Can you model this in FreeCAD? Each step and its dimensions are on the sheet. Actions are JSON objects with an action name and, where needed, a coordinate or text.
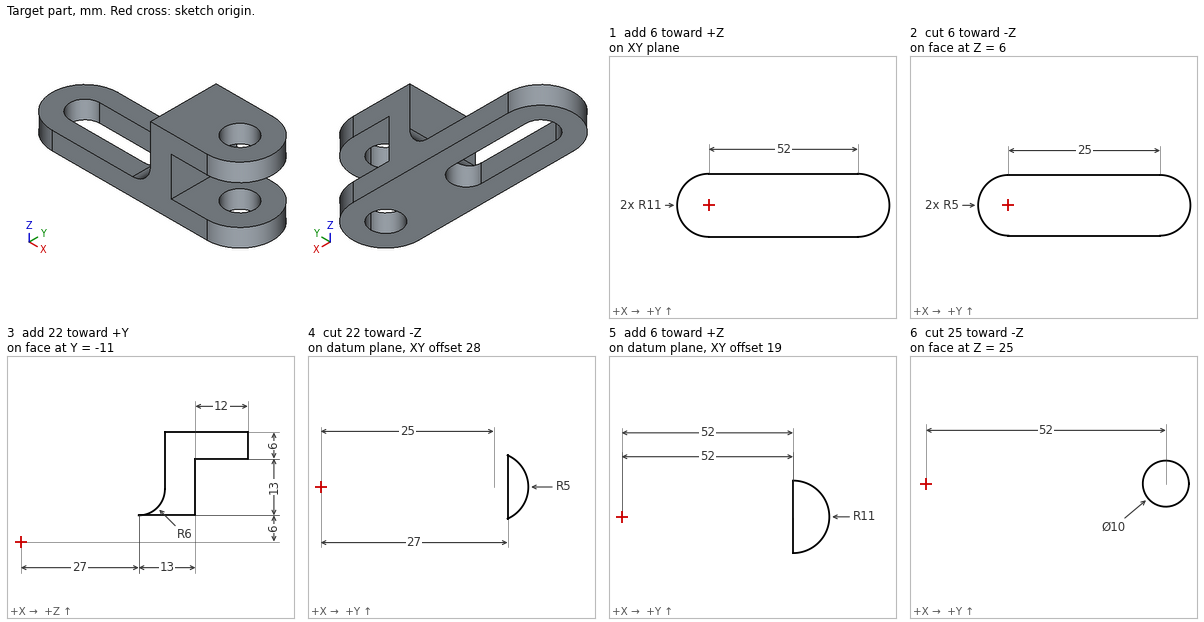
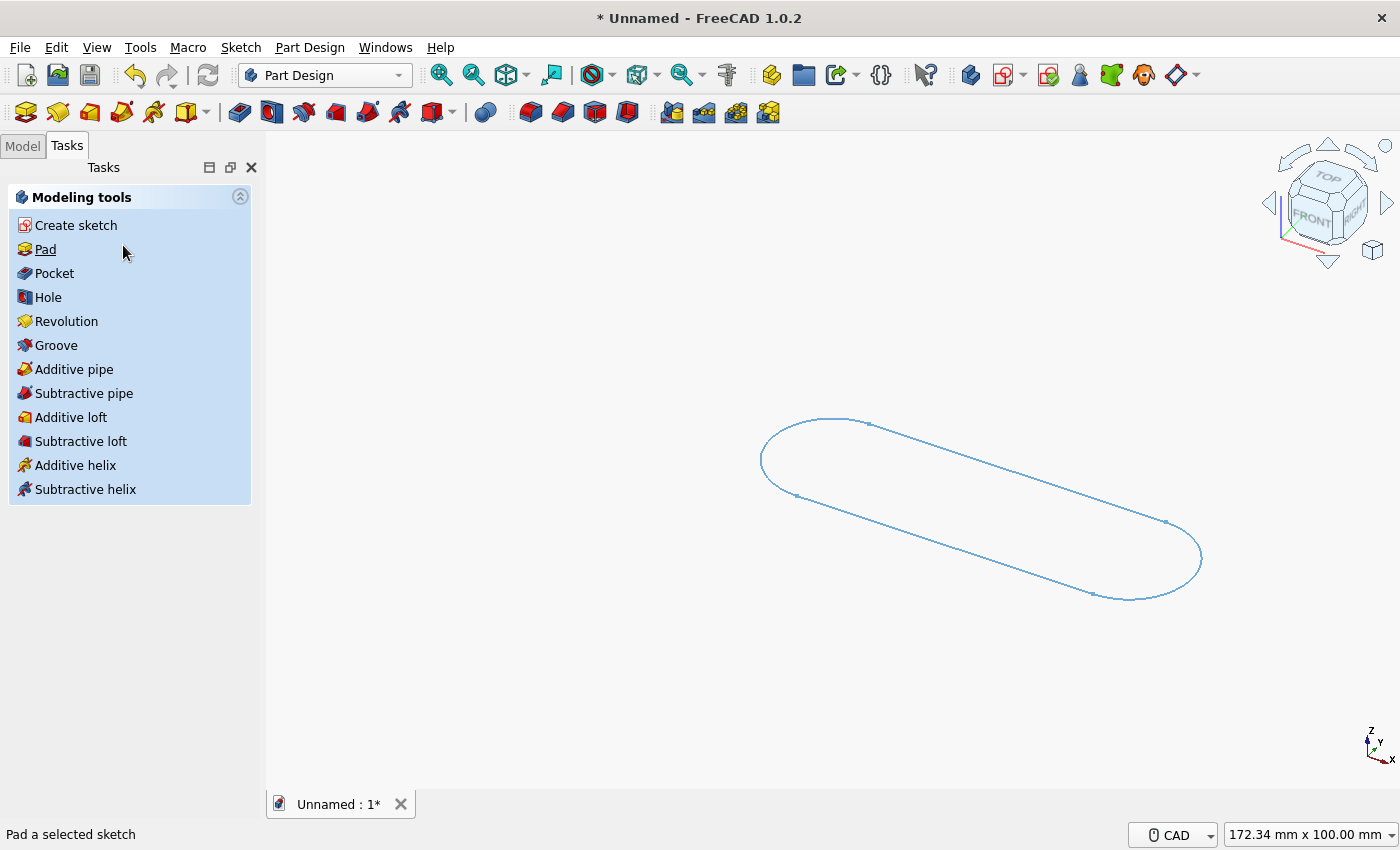
{"action": "left_click", "coordinate": [26, 112]}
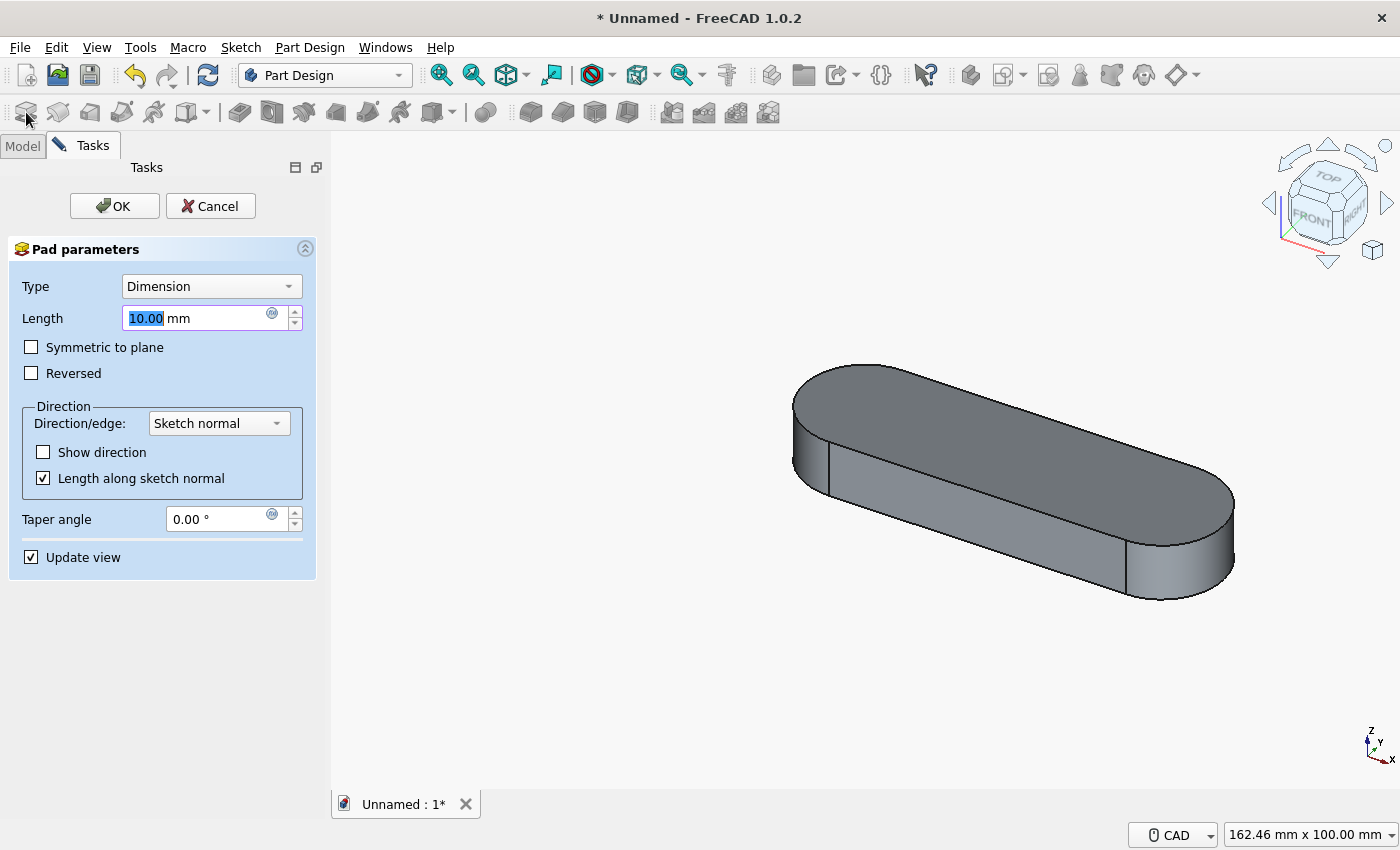
{"action": "type", "text": "6"}
{"action": "key", "text": "Tab"}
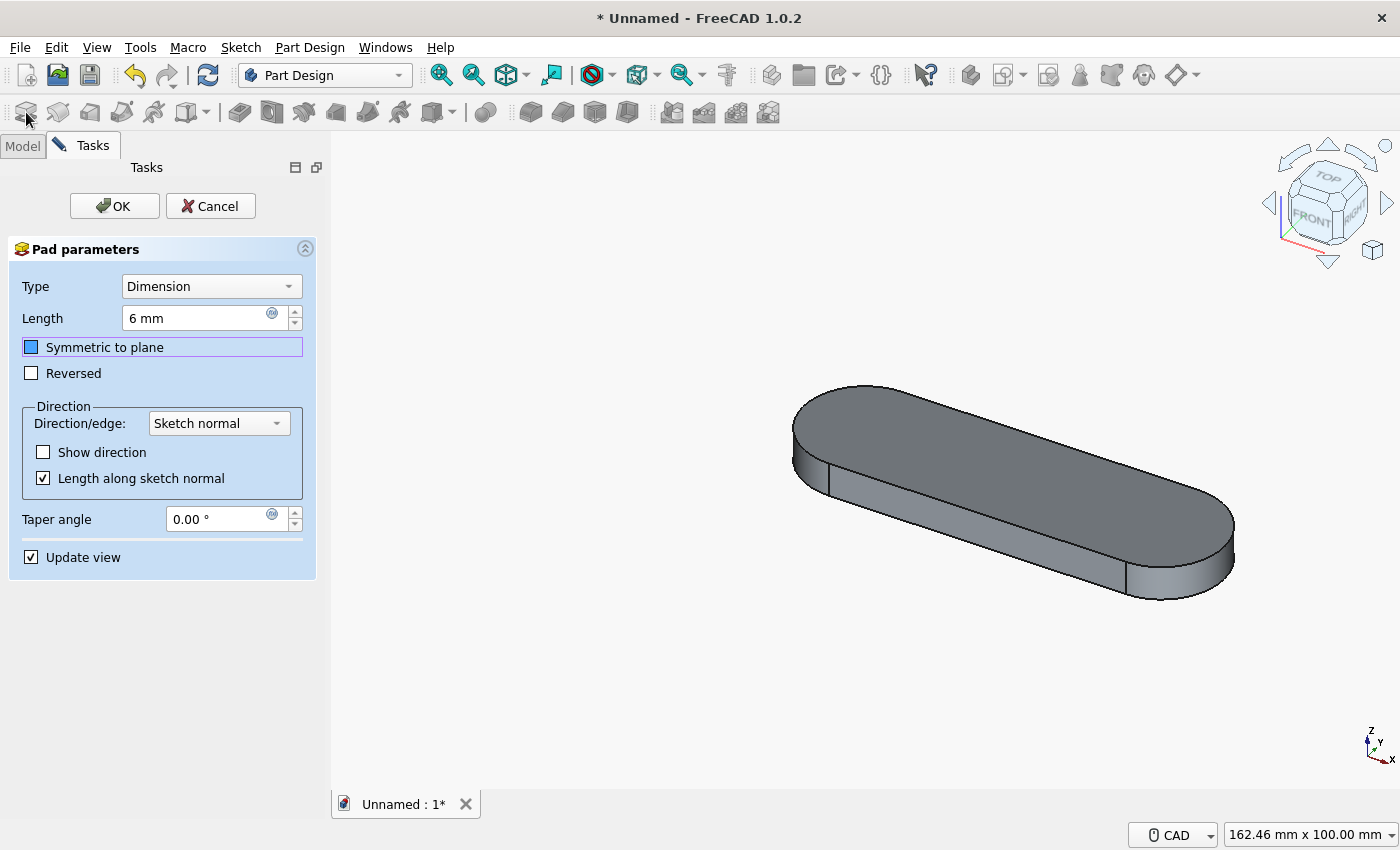
{"action": "left_click", "coordinate": [115, 206]}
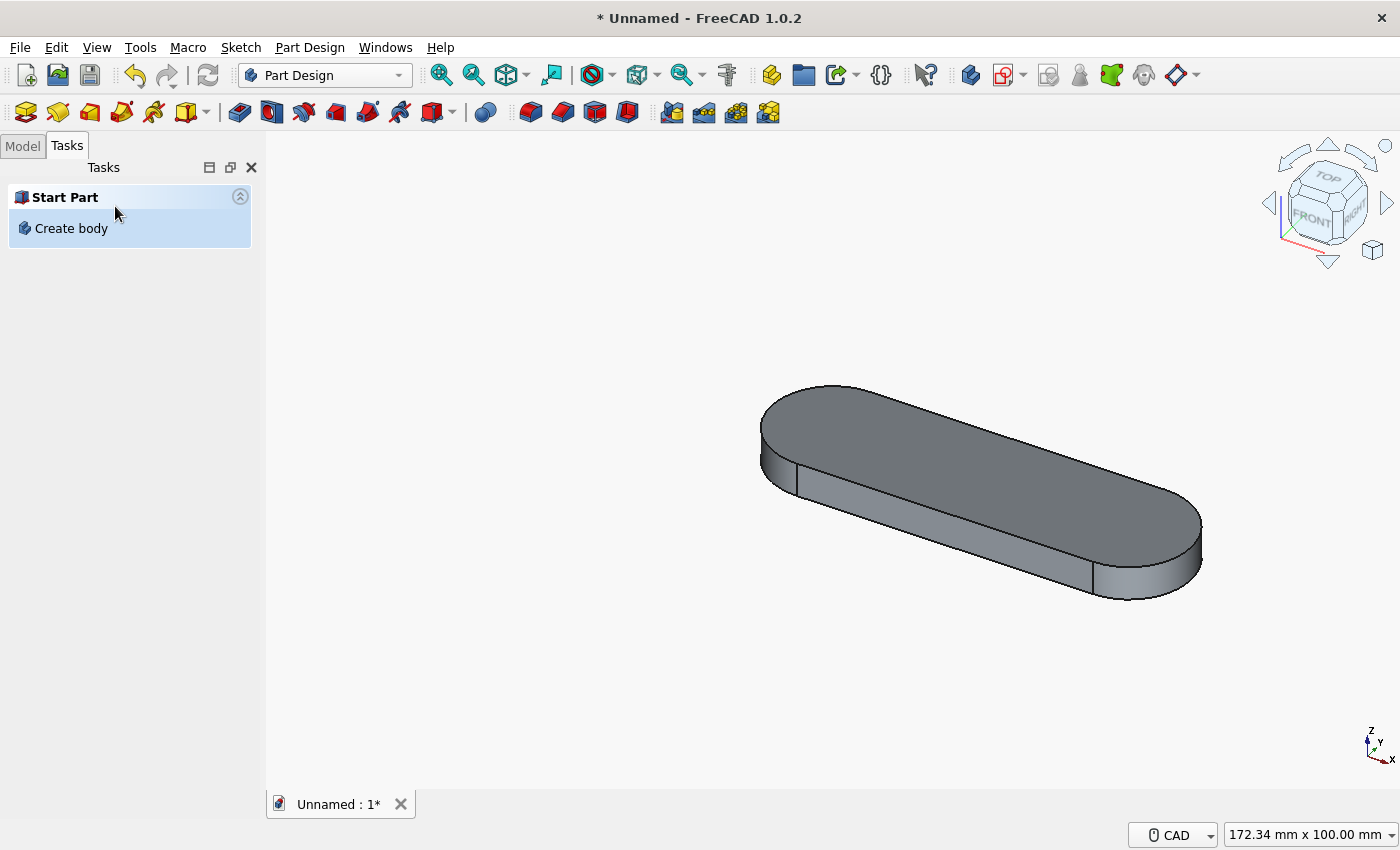
{"action": "left_click", "coordinate": [442, 76]}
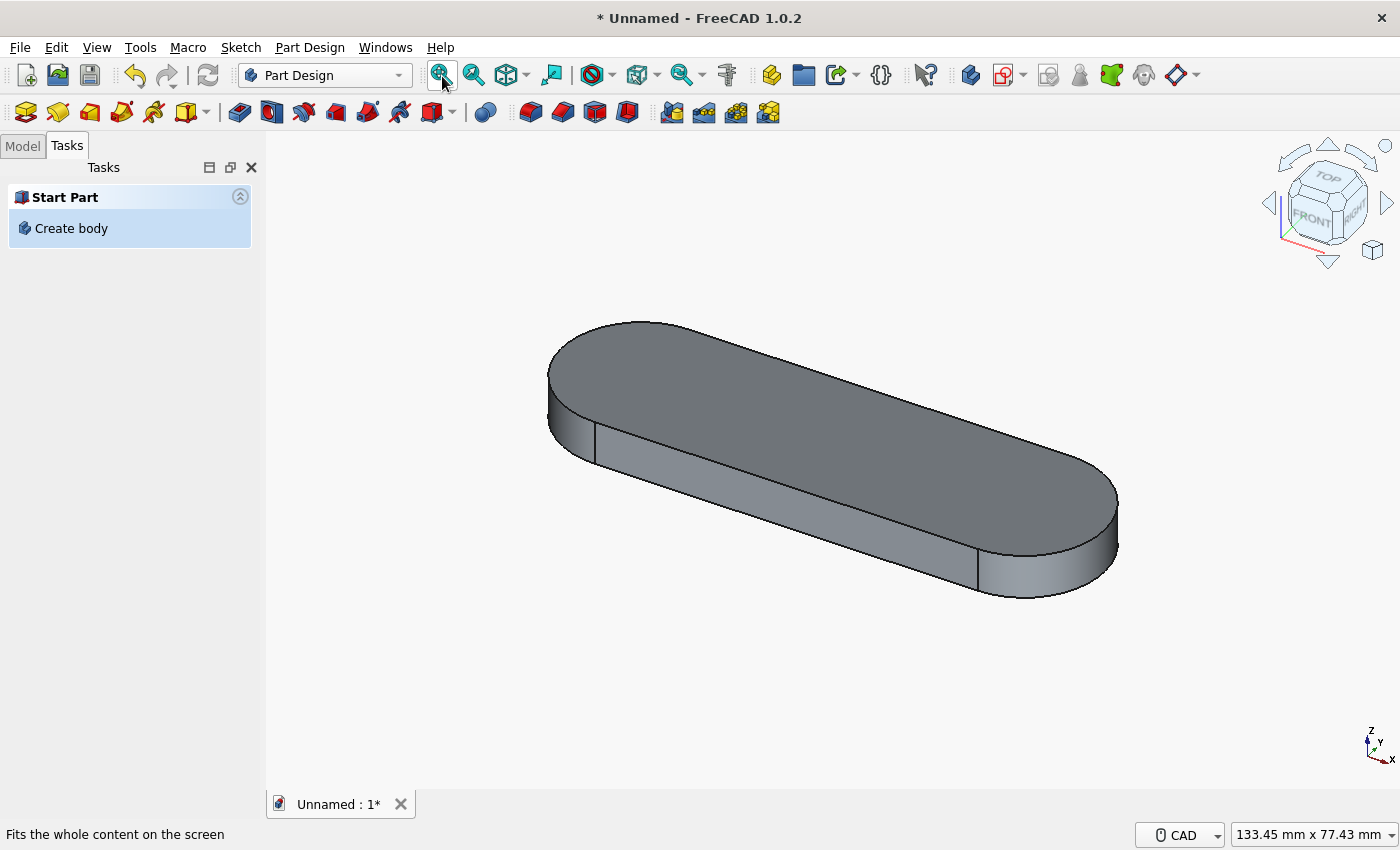
{"action": "left_click", "coordinate": [989, 490]}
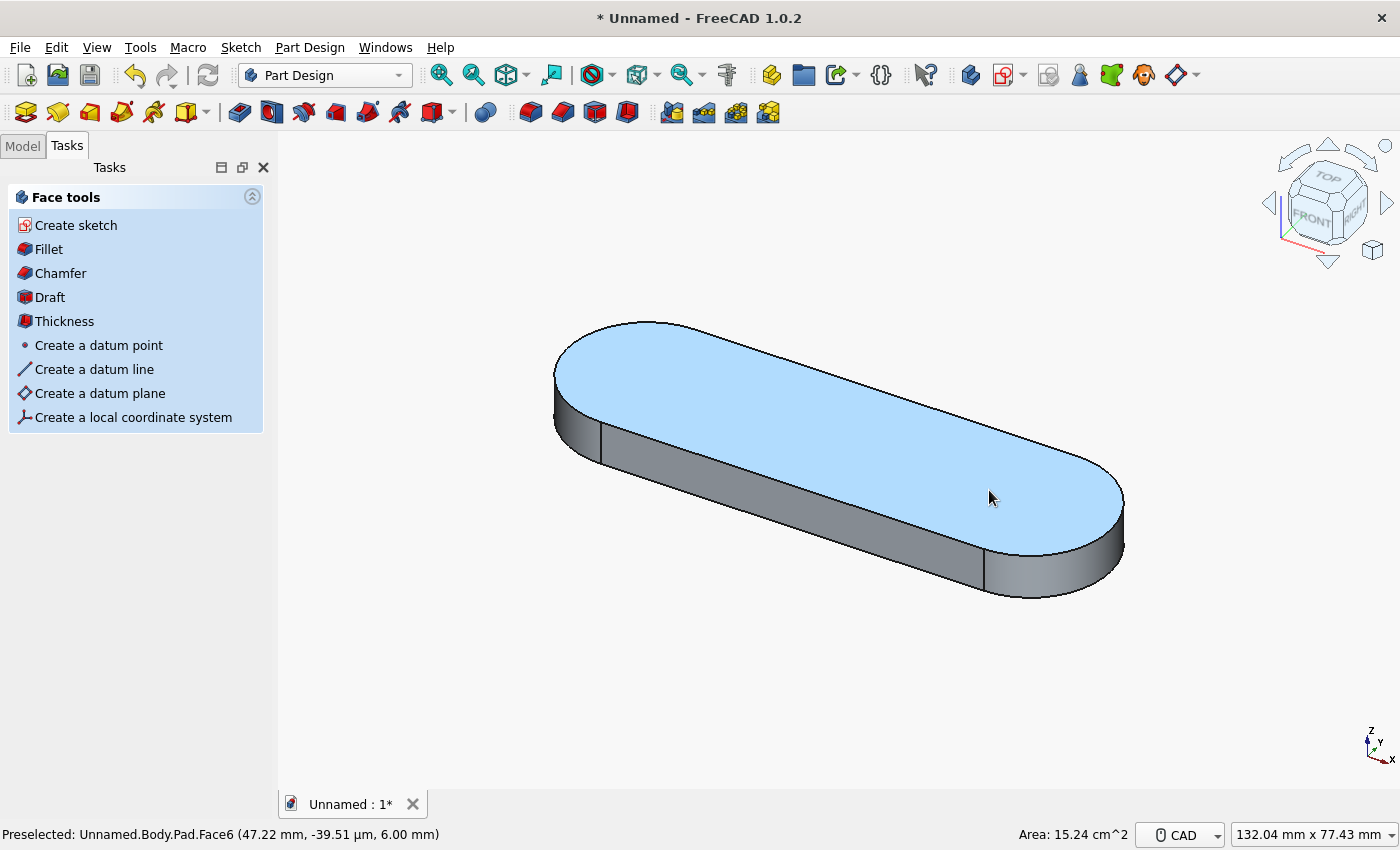
{"action": "left_click", "coordinate": [1004, 76]}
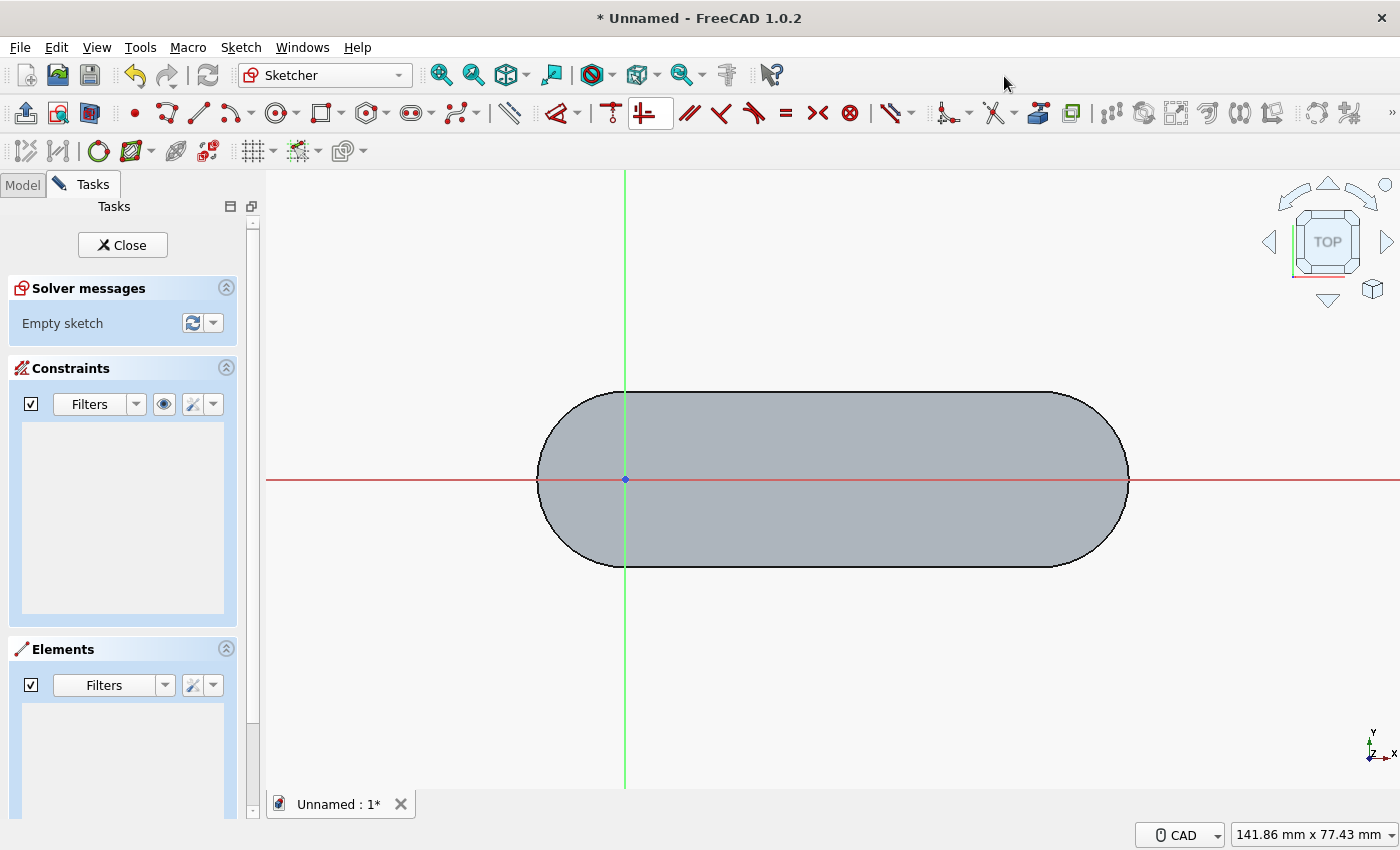
{"action": "scroll", "coordinate": [693, 480], "scroll_direction": "up", "scroll_amount": 4}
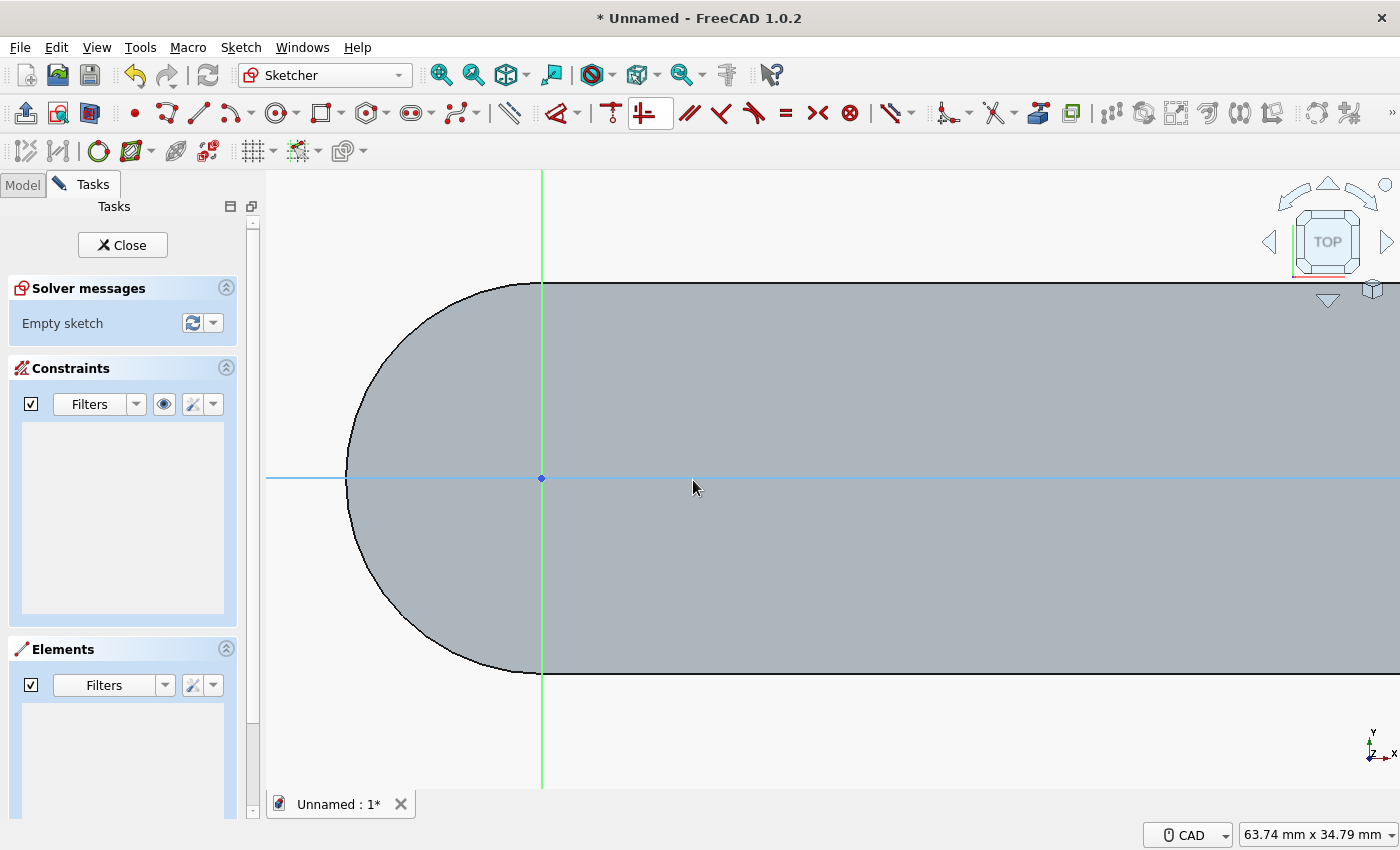
{"action": "left_click", "coordinate": [412, 114]}